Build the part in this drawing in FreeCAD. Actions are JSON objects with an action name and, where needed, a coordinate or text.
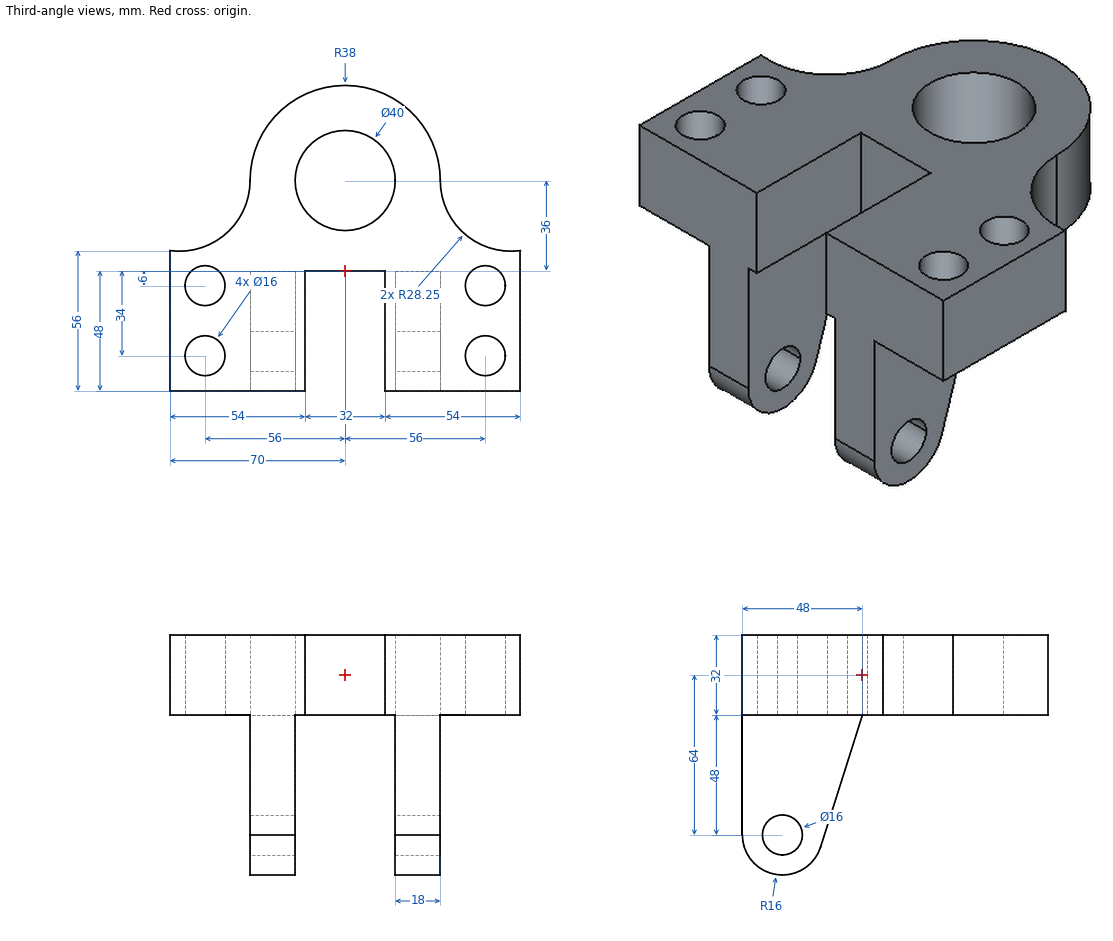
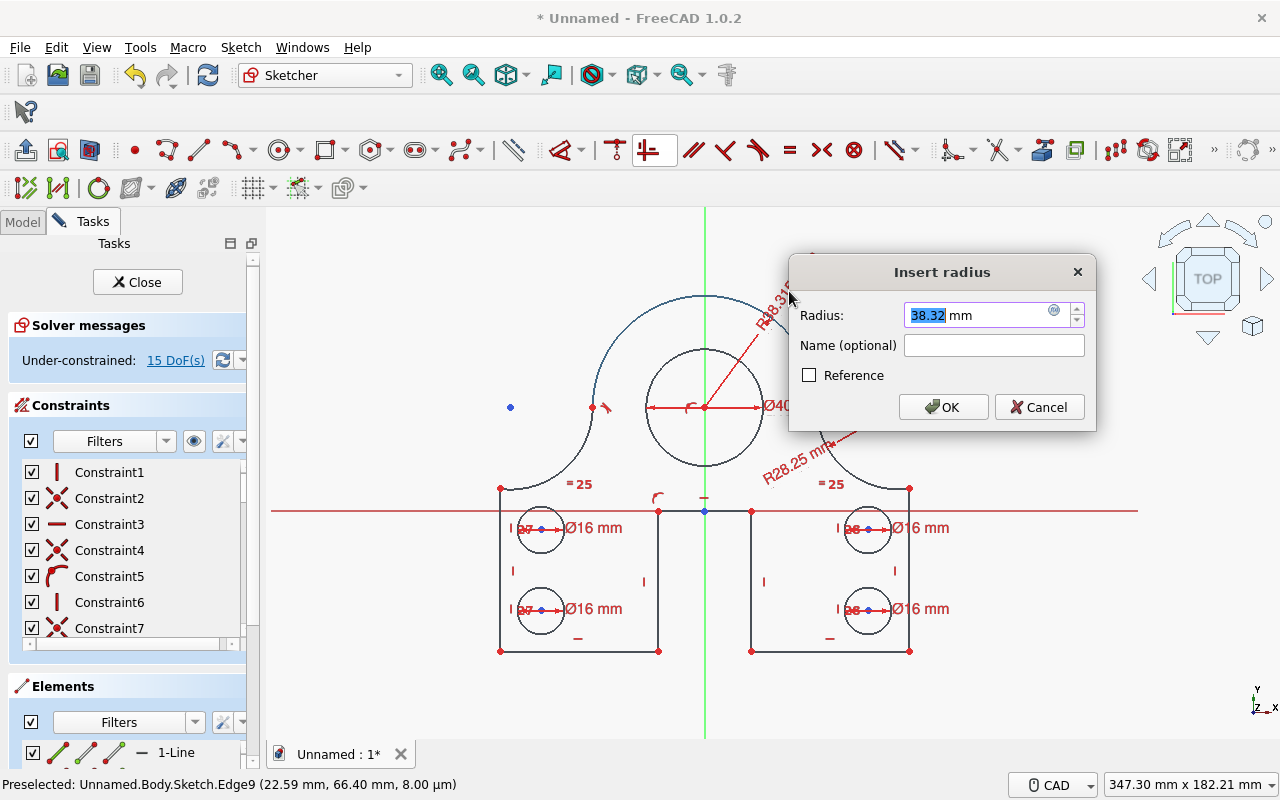
{"action": "type", "text": "38"}
{"action": "key", "text": "Return"}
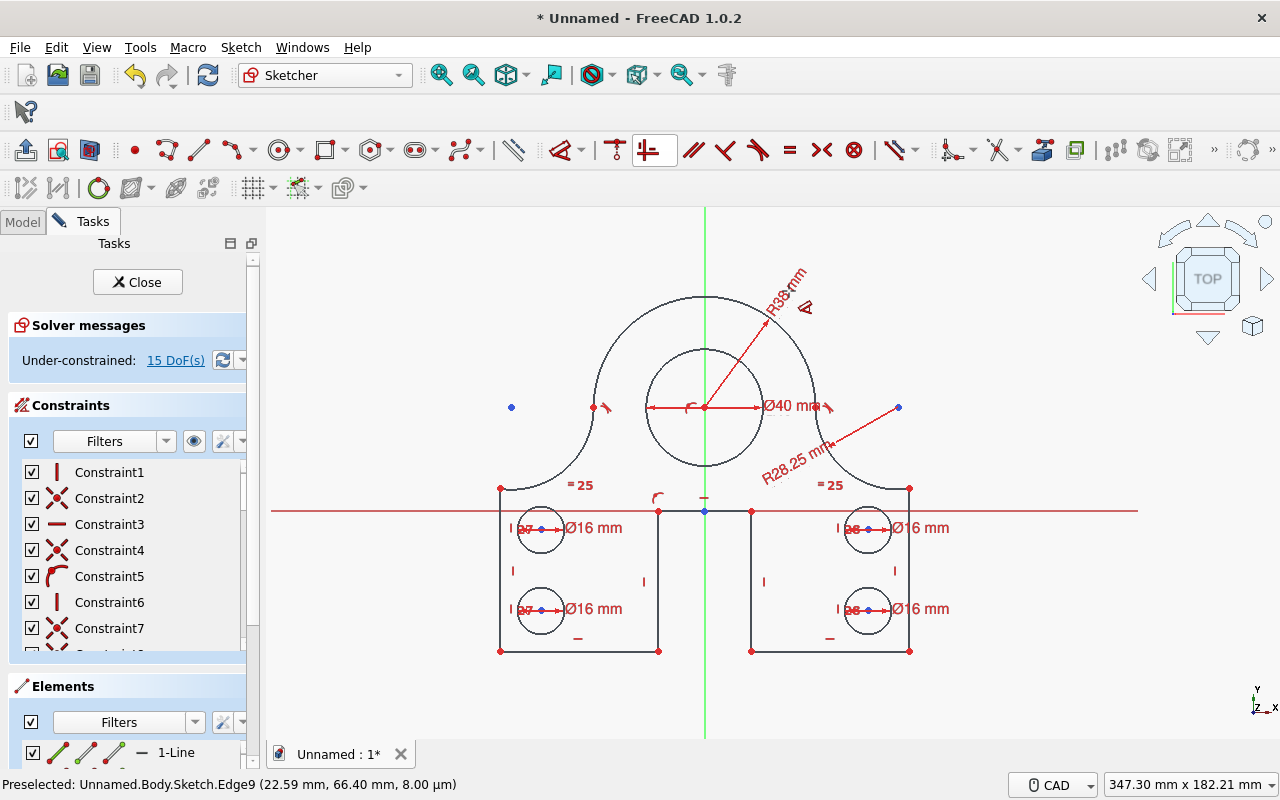
{"action": "scroll", "coordinate": [541, 530], "scroll_direction": "up", "scroll_amount": 5}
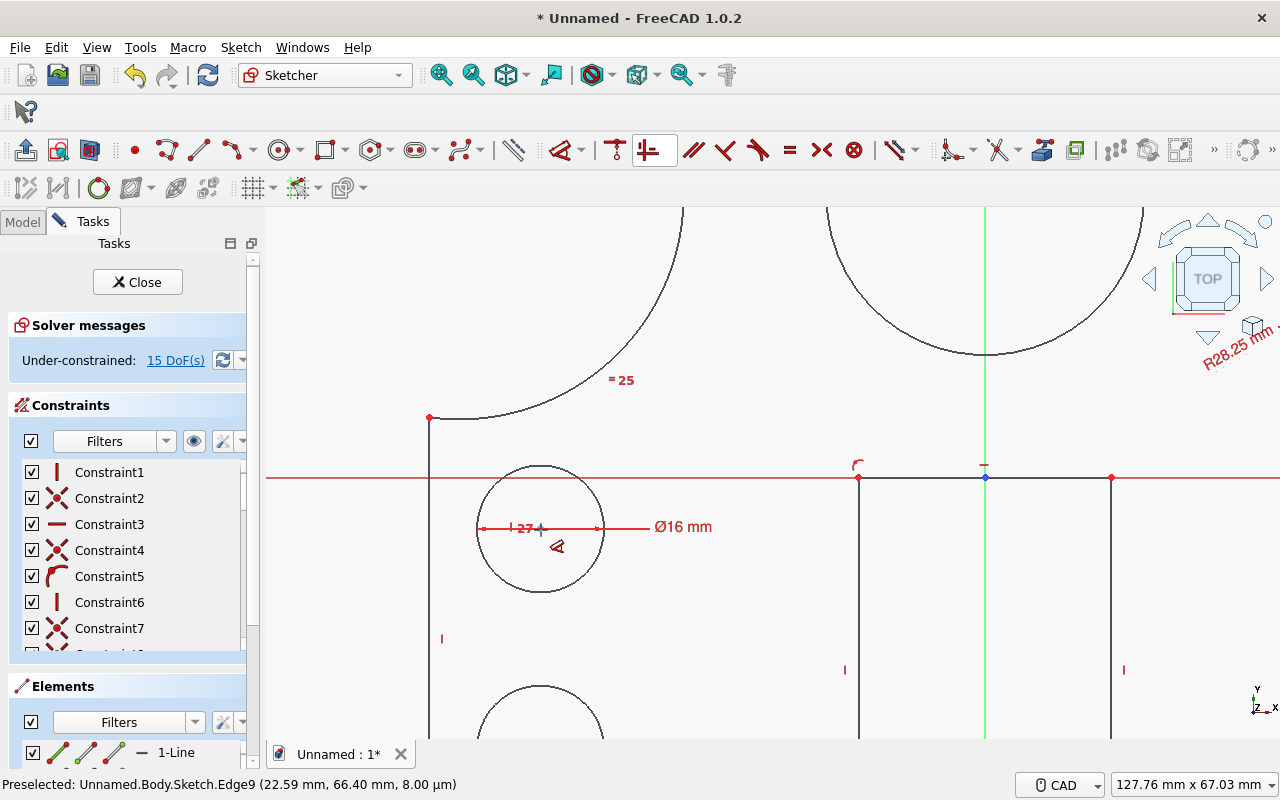
{"action": "left_click", "coordinate": [541, 529]}
{"action": "left_click", "coordinate": [507, 503]}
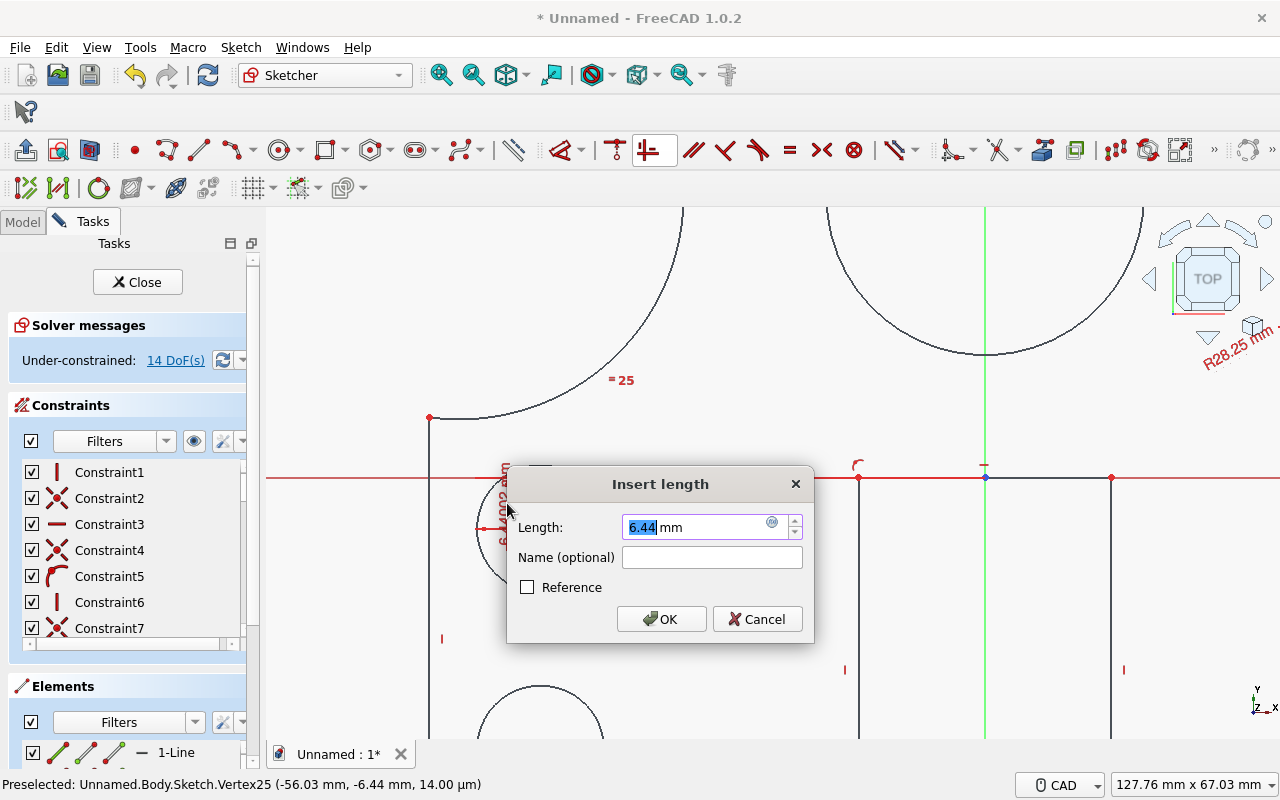
{"action": "type", "text": "6"}
{"action": "key", "text": "Return"}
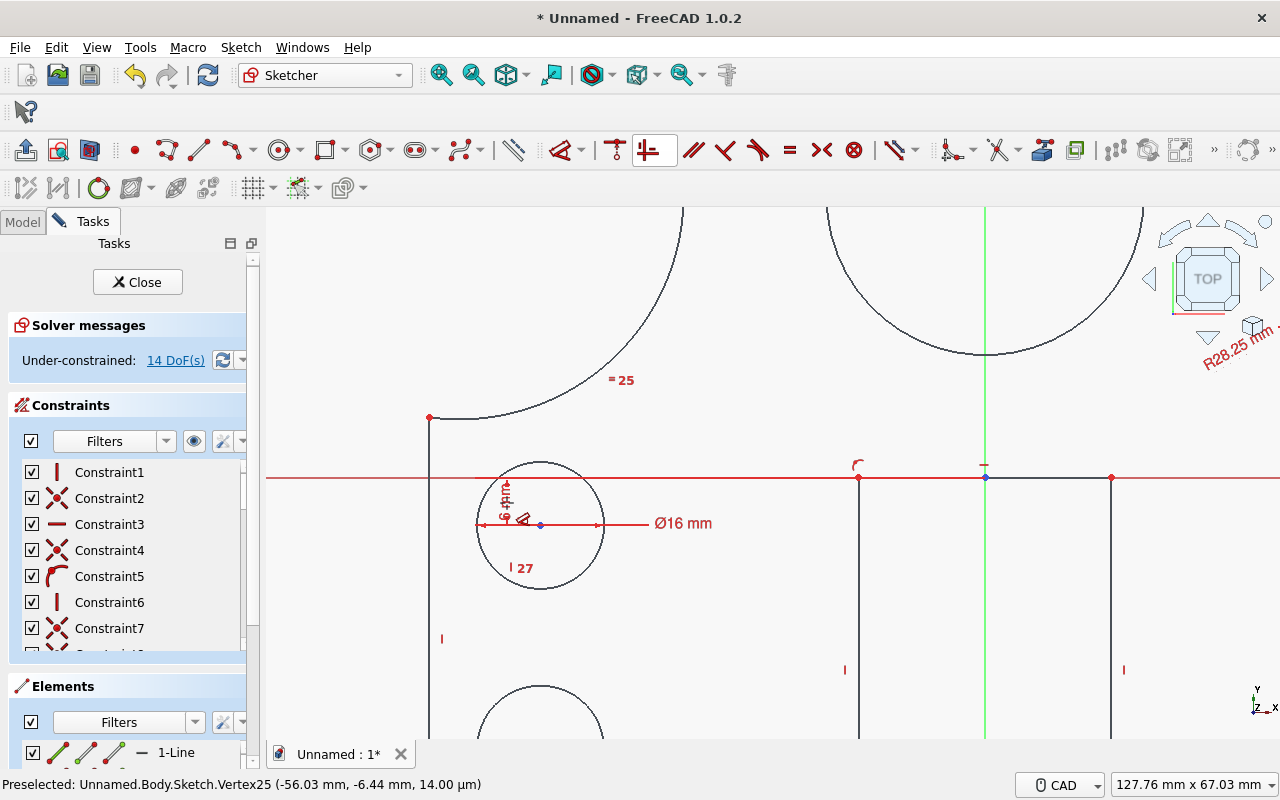
{"action": "scroll", "coordinate": [541, 530], "scroll_direction": "down", "scroll_amount": 5}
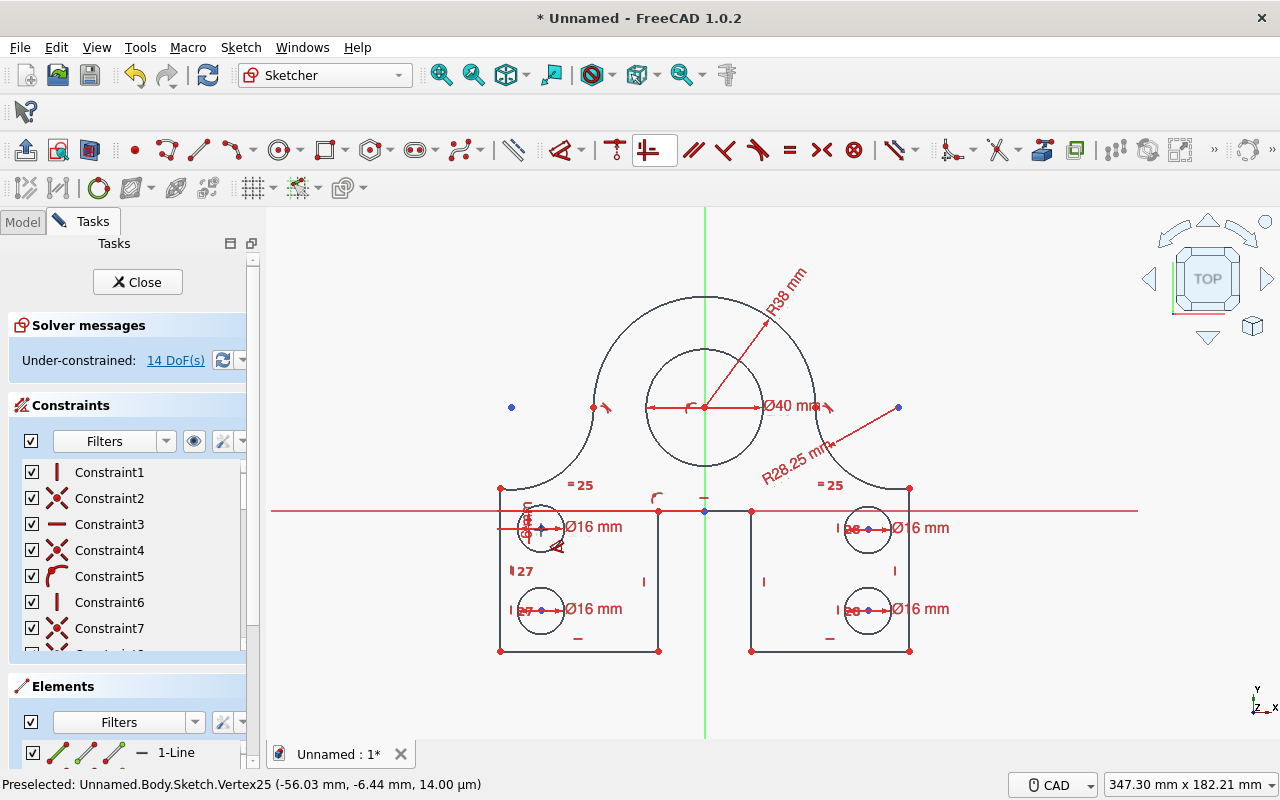
{"action": "scroll", "coordinate": [868, 530], "scroll_direction": "up", "scroll_amount": 5}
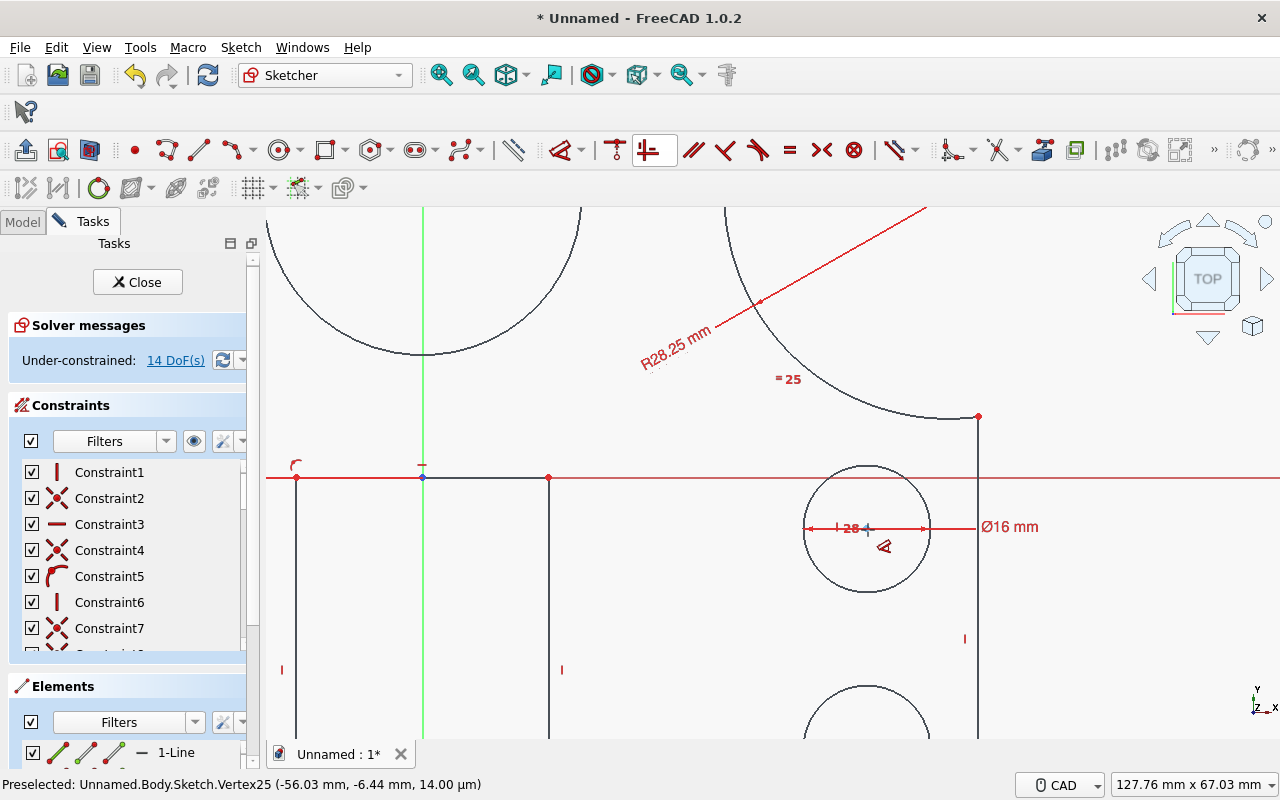
{"action": "left_click", "coordinate": [867, 529]}
{"action": "left_click", "coordinate": [901, 503]}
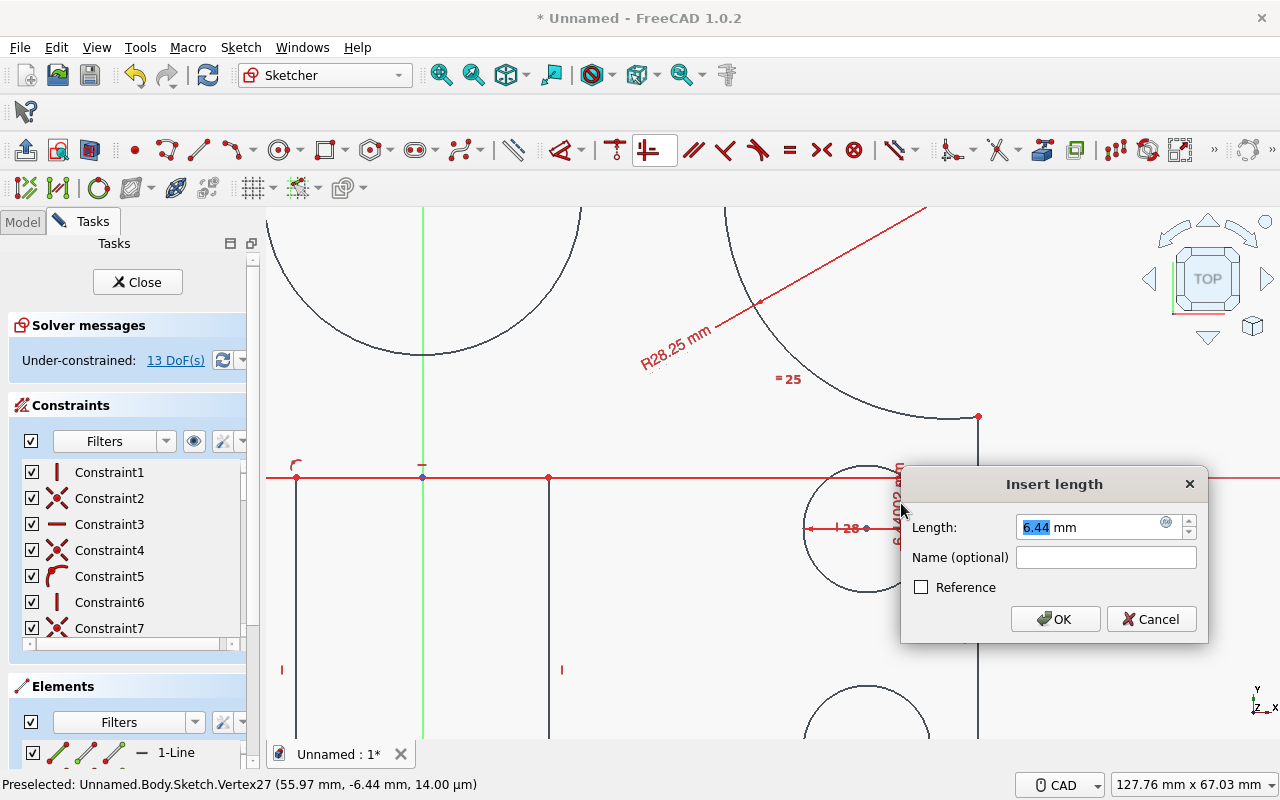
{"action": "type", "text": "6"}
{"action": "key", "text": "Return"}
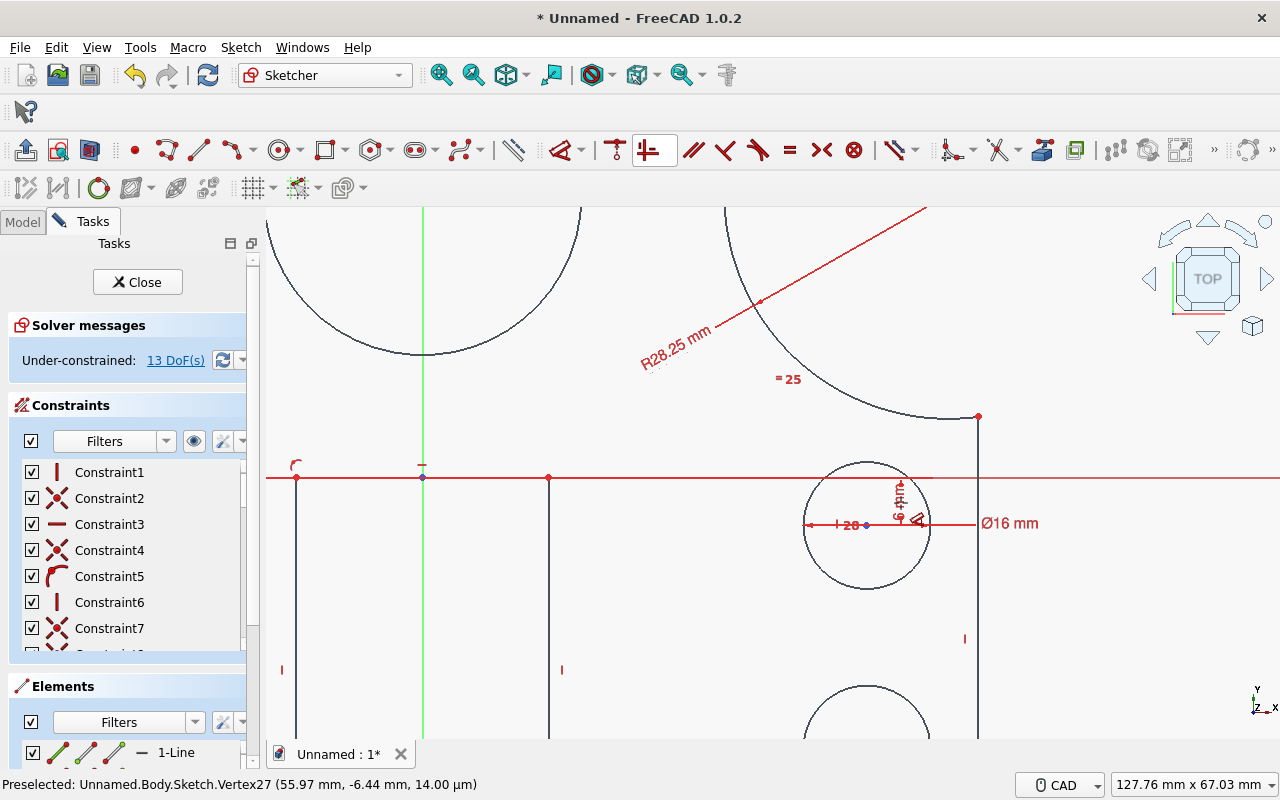
{"action": "scroll", "coordinate": [868, 530], "scroll_direction": "down", "scroll_amount": 5}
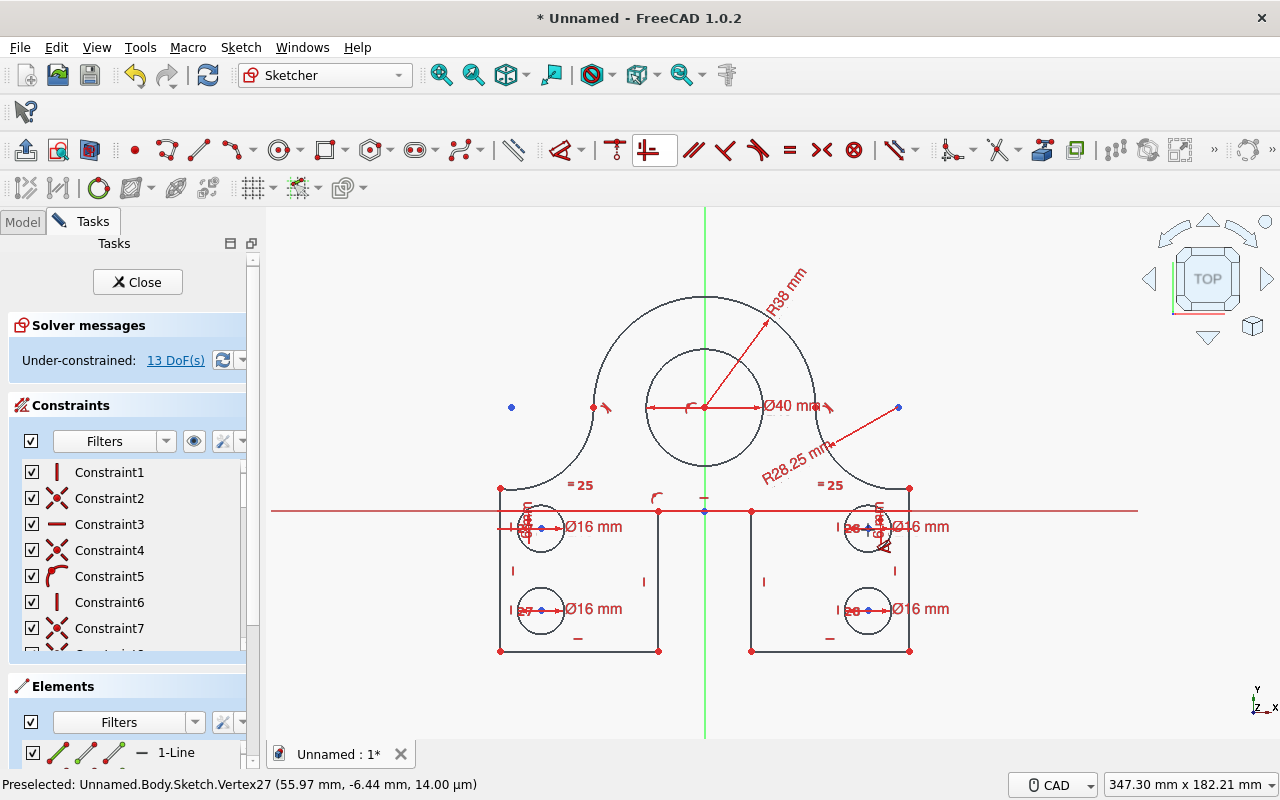
{"action": "left_click", "coordinate": [500, 538]}
{"action": "left_click", "coordinate": [466, 570]}